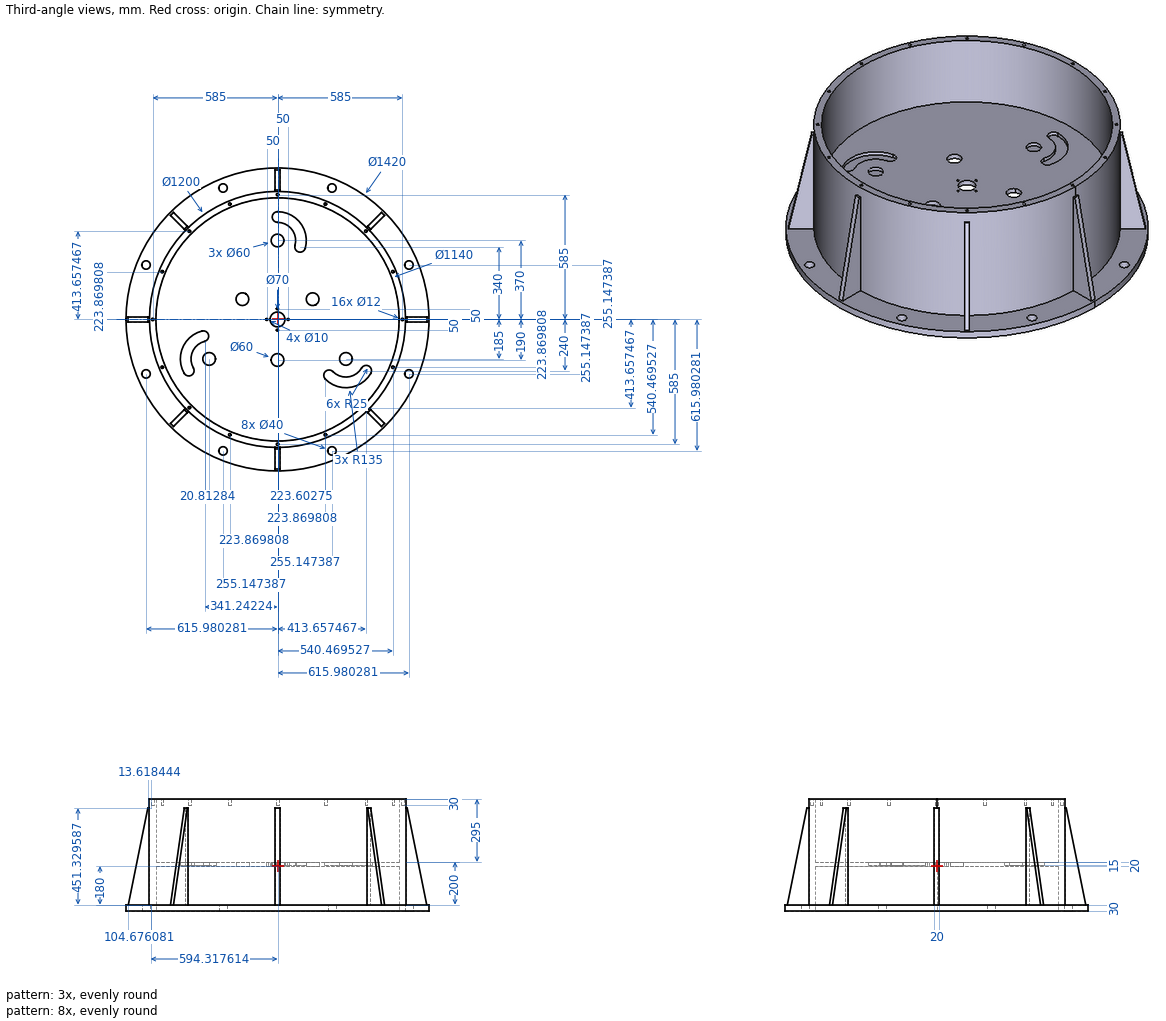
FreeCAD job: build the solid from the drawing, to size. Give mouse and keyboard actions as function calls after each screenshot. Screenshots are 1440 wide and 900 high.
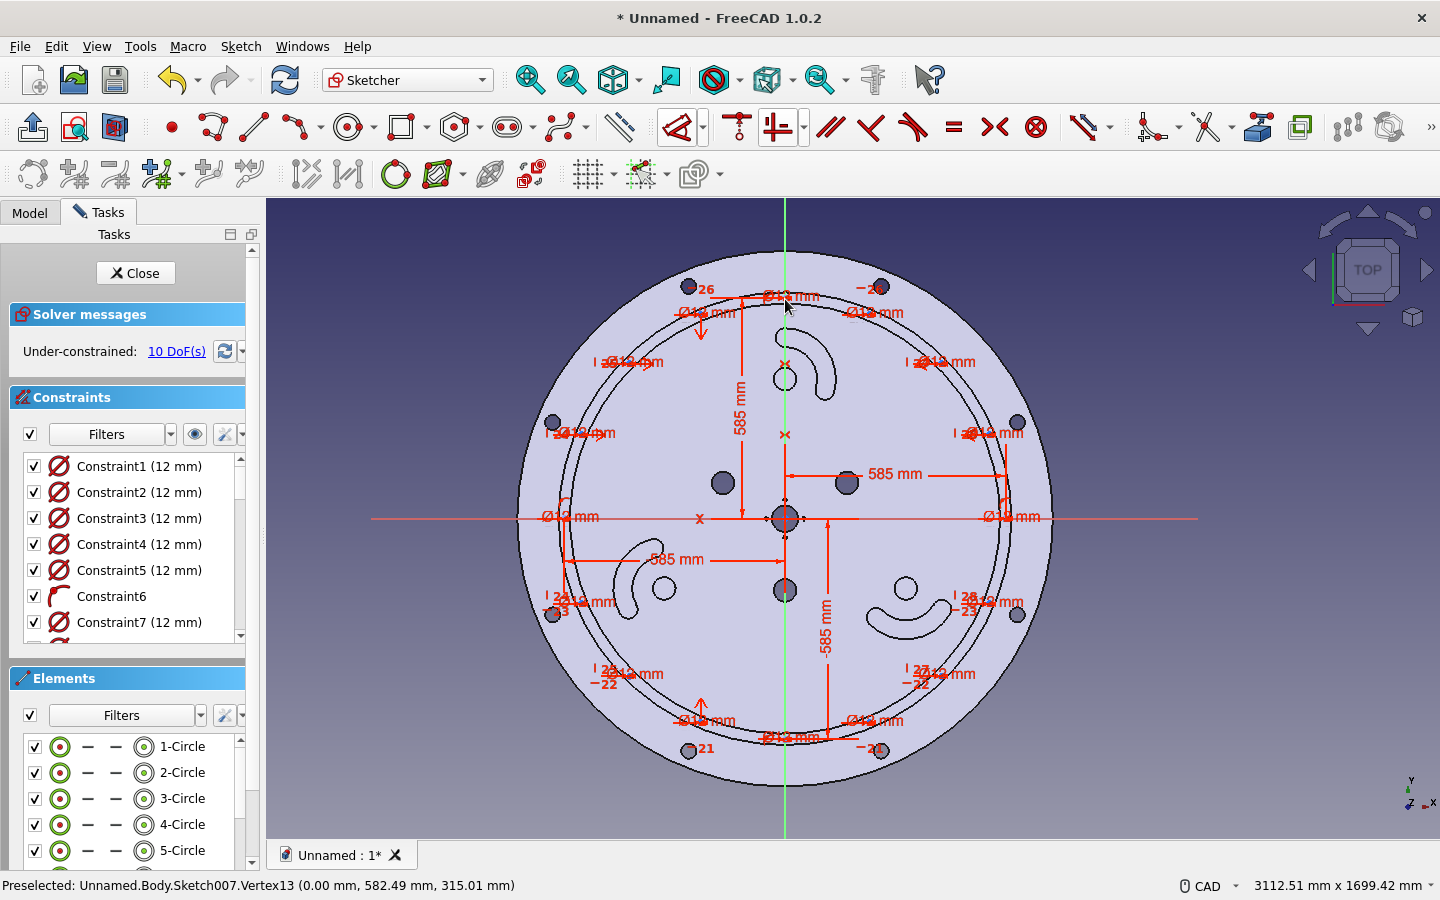
click(989, 604)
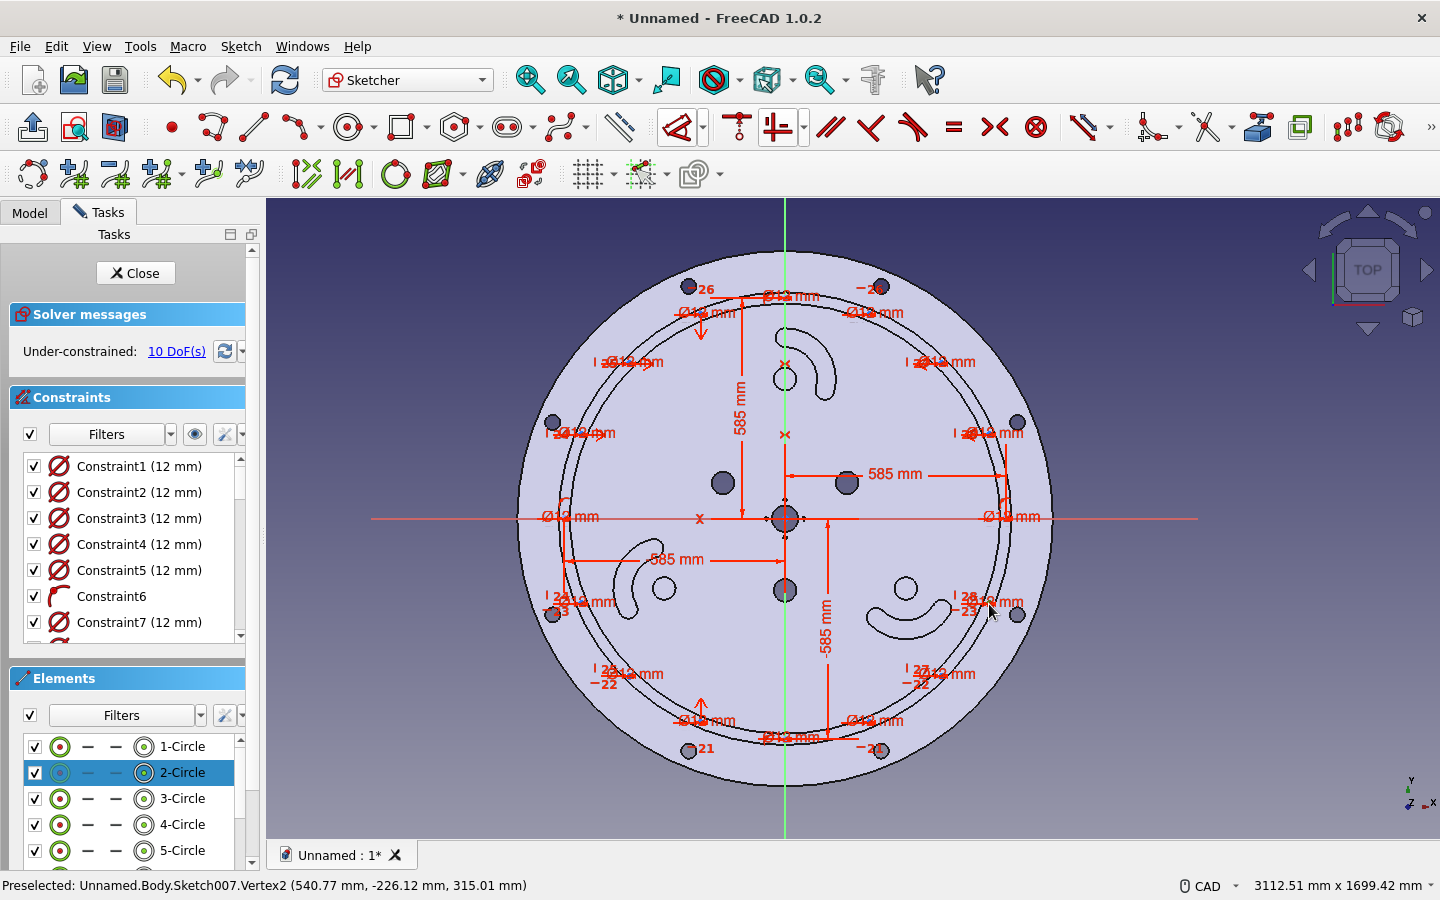
key(l)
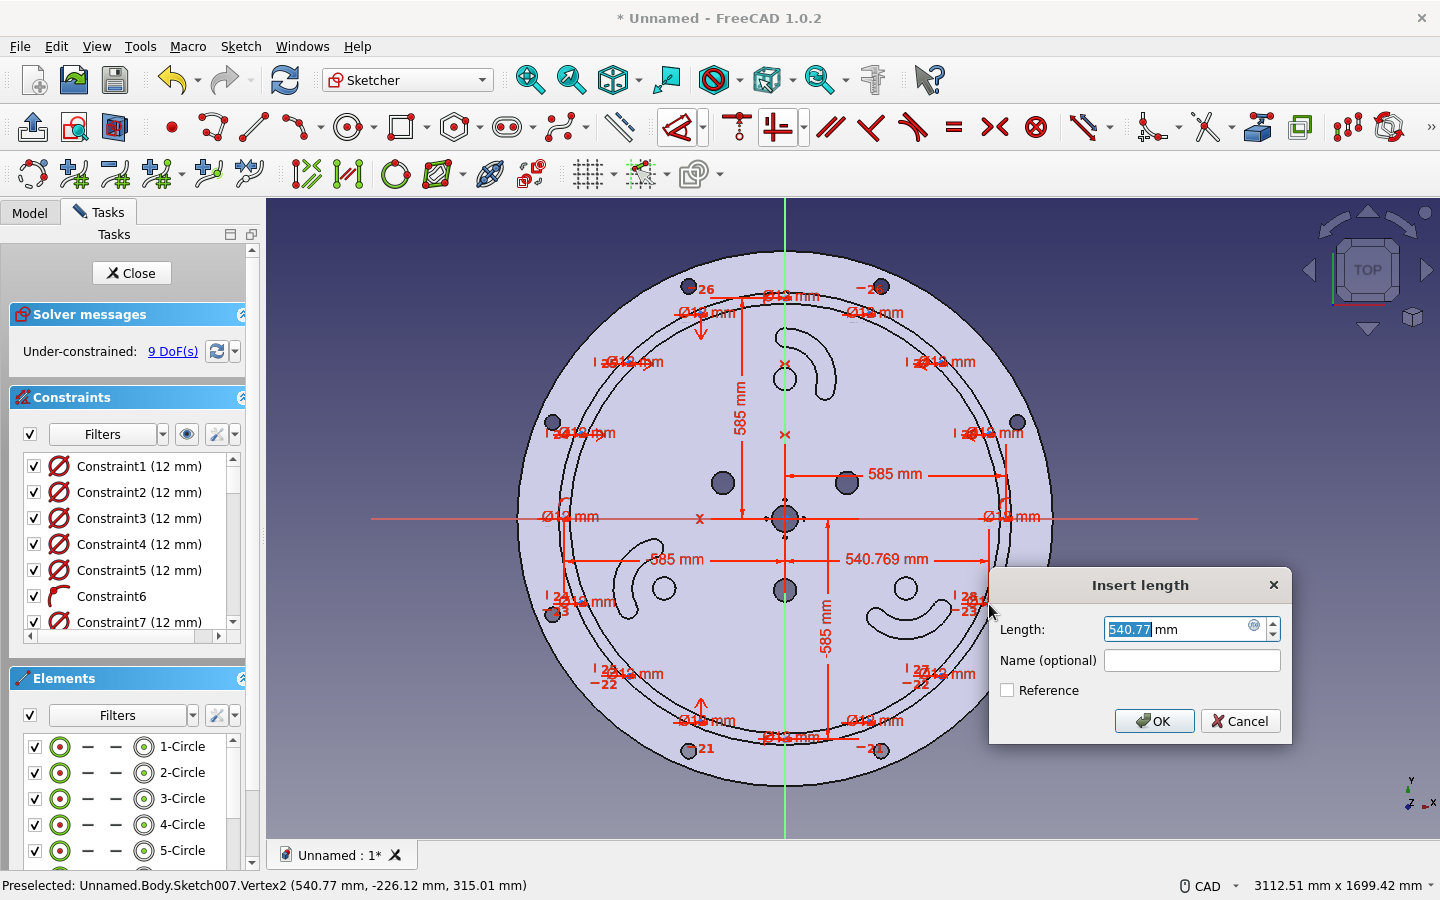
text(540.469527)
key(Return)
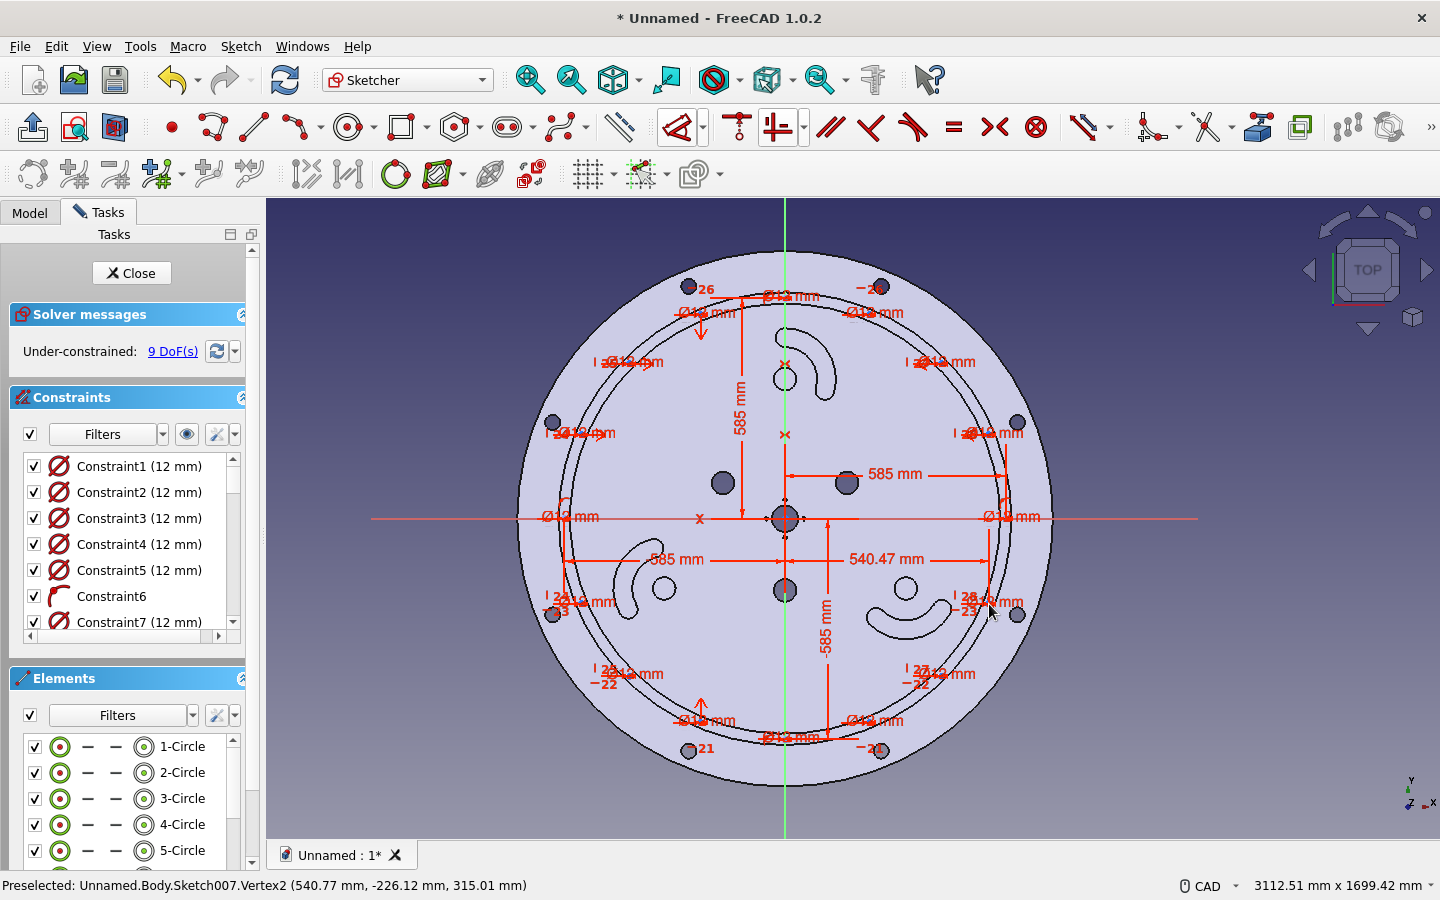
click(989, 604)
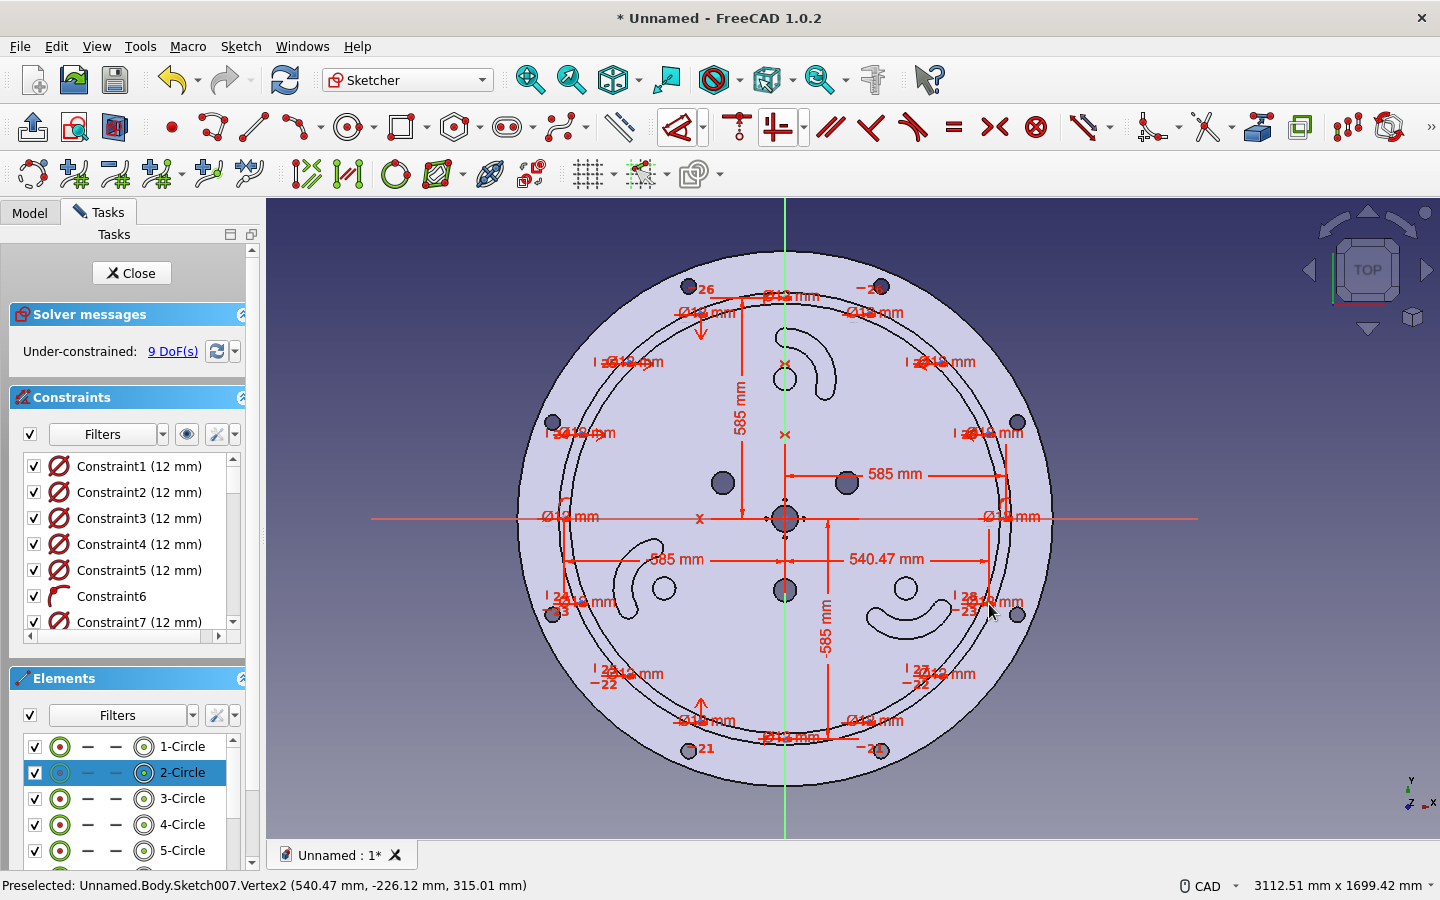
key(i)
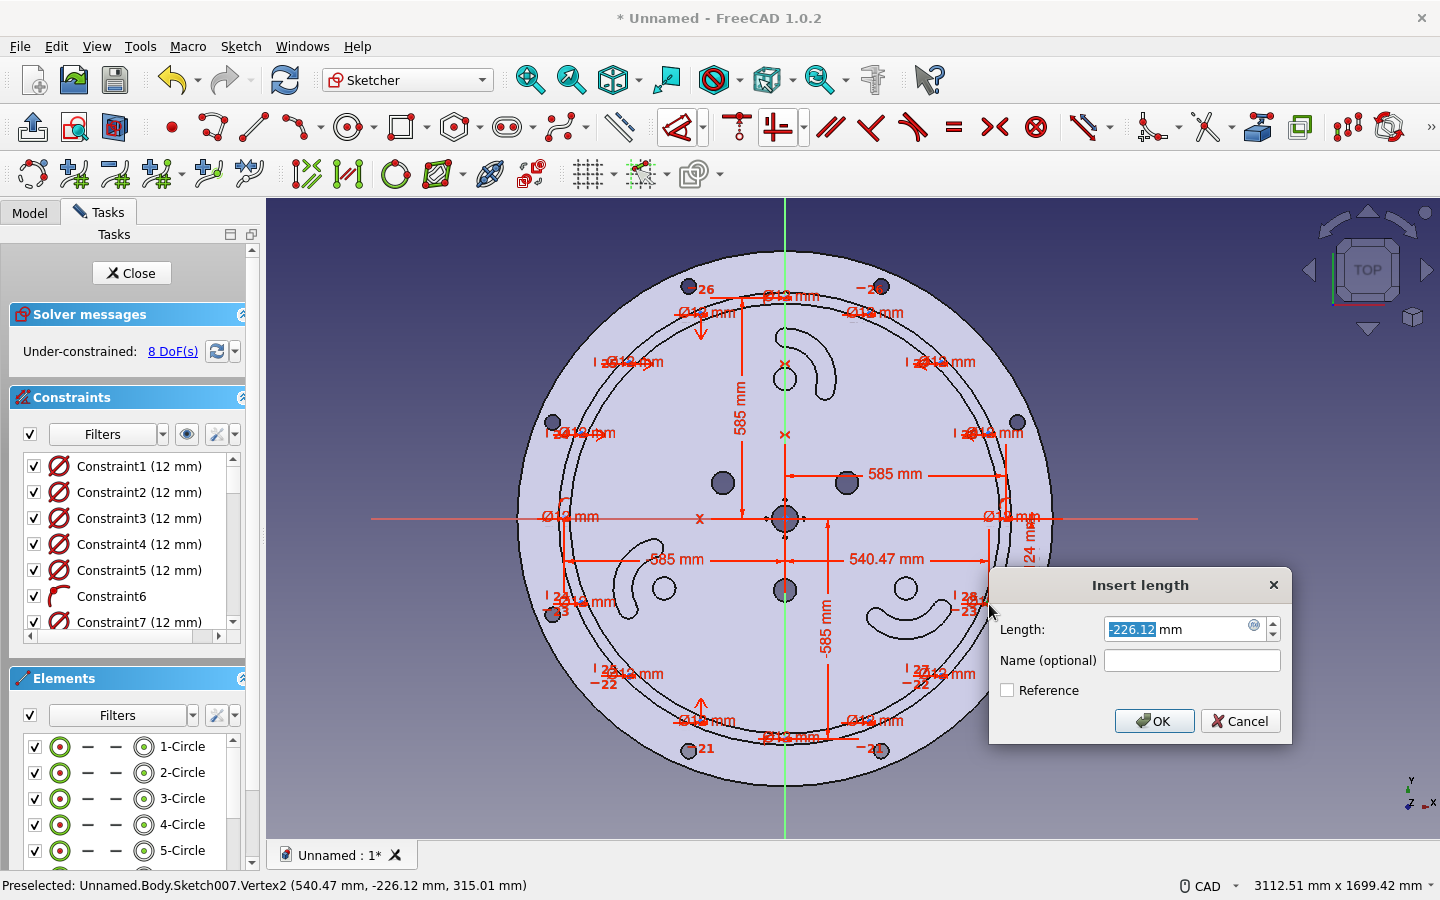
text(-223.869808)
key(Return)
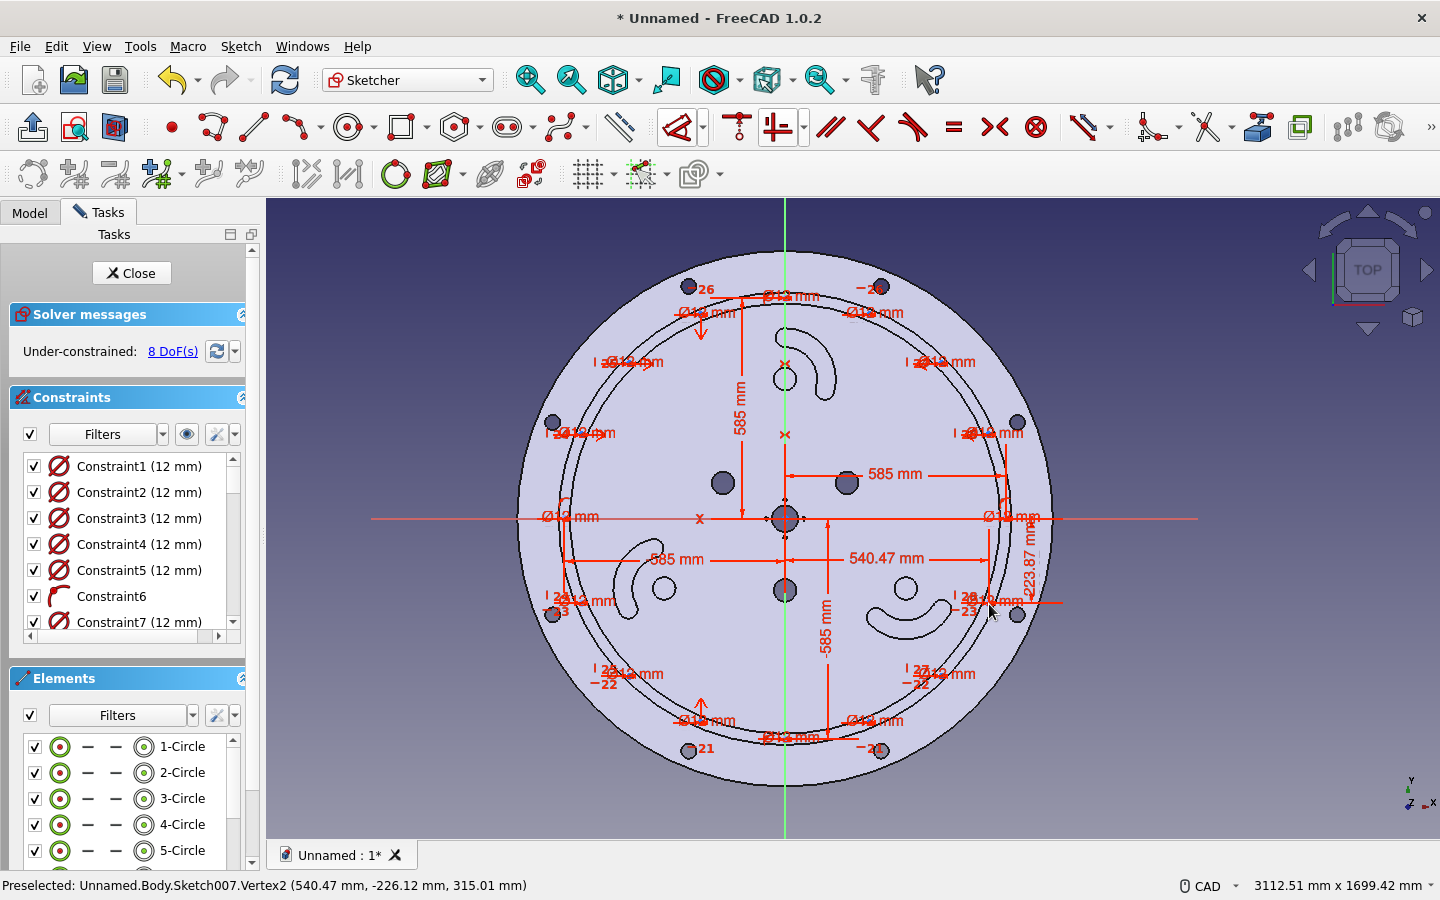
click(941, 676)